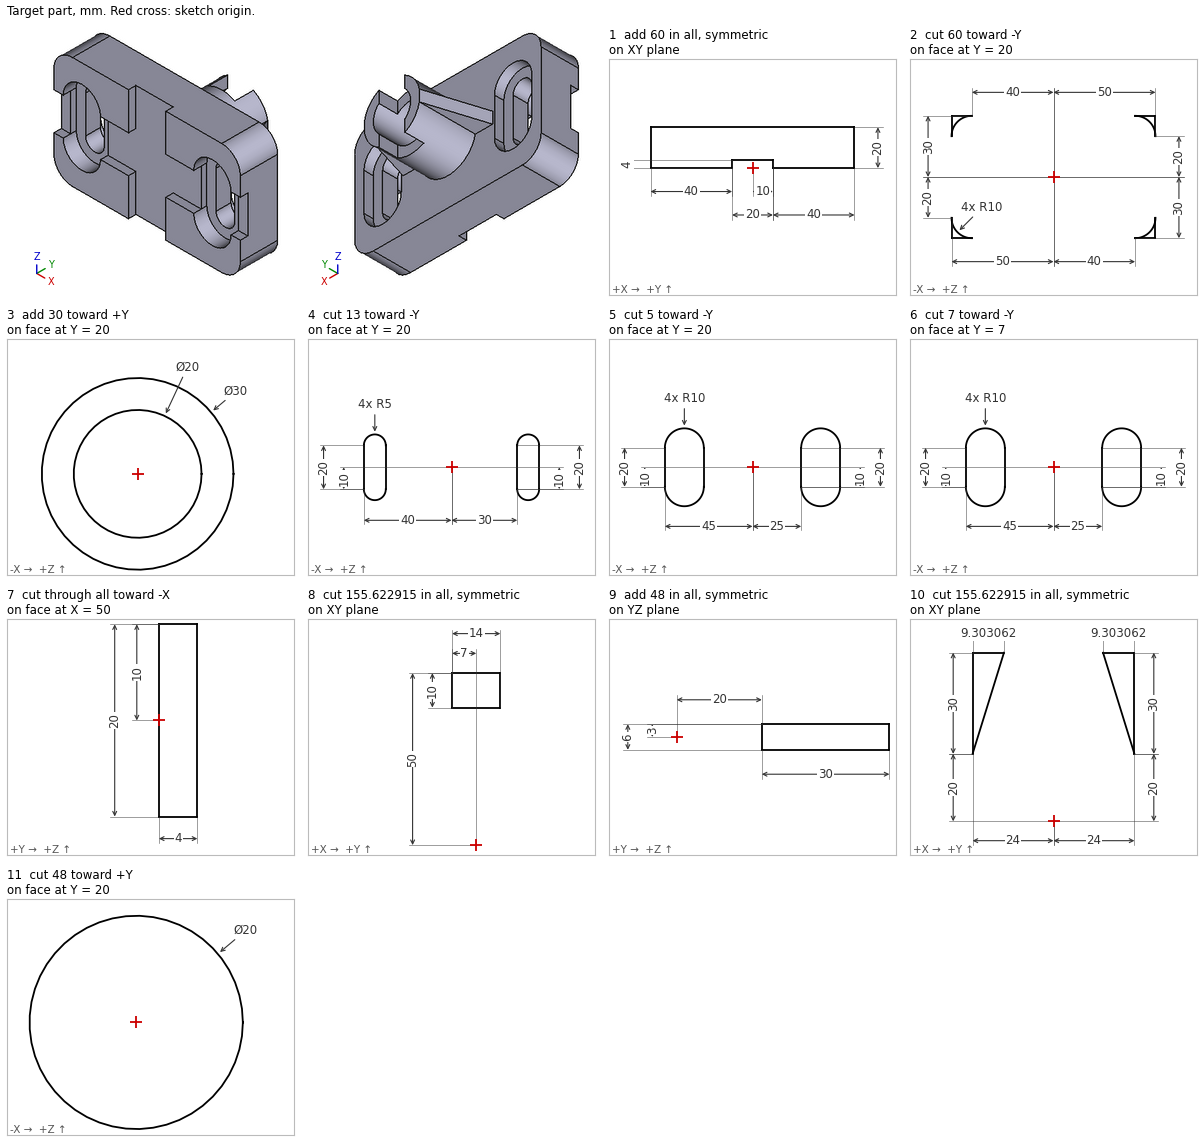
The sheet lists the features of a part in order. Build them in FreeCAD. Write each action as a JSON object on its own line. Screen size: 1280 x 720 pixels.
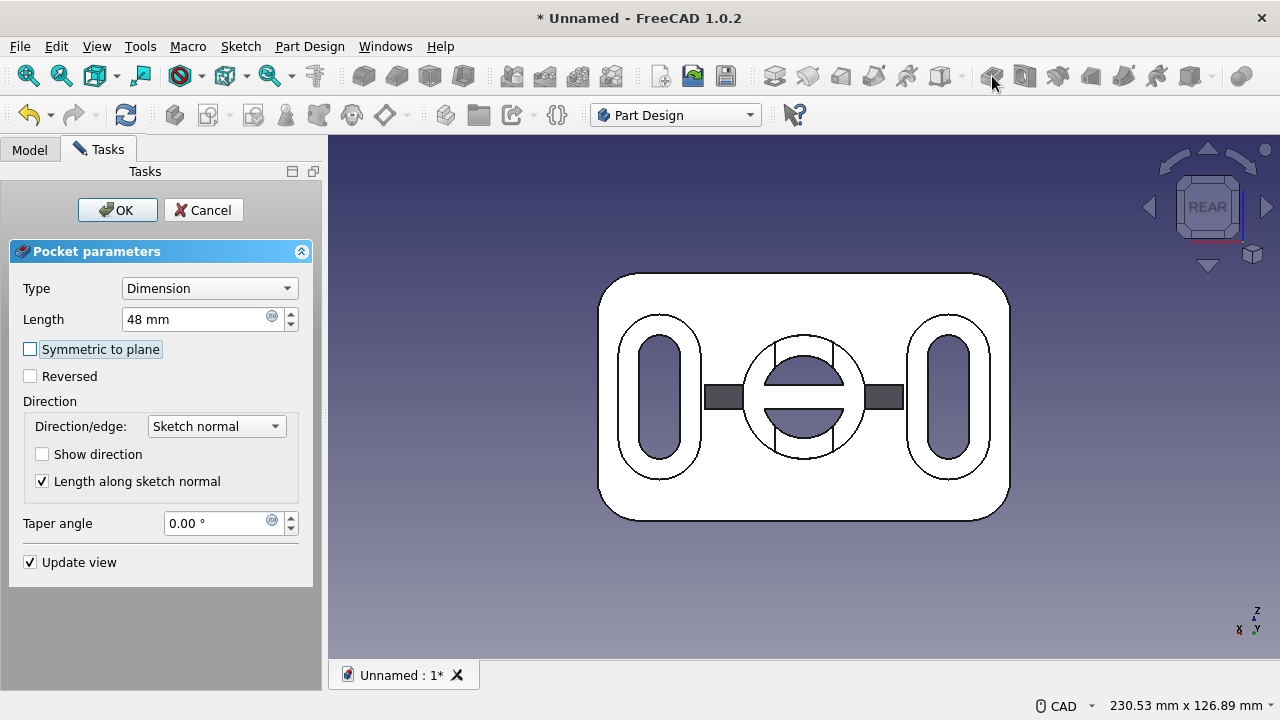
{"action": "left_click", "coordinate": [31, 376]}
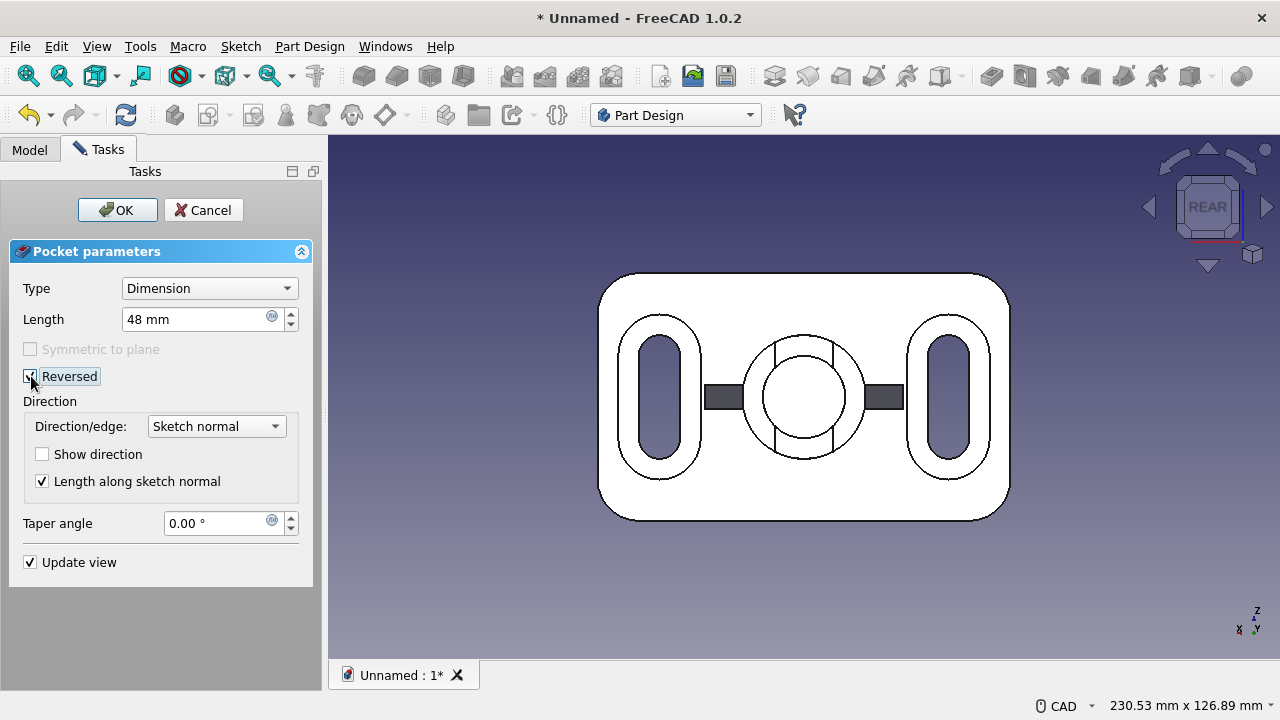
{"action": "left_click", "coordinate": [118, 210]}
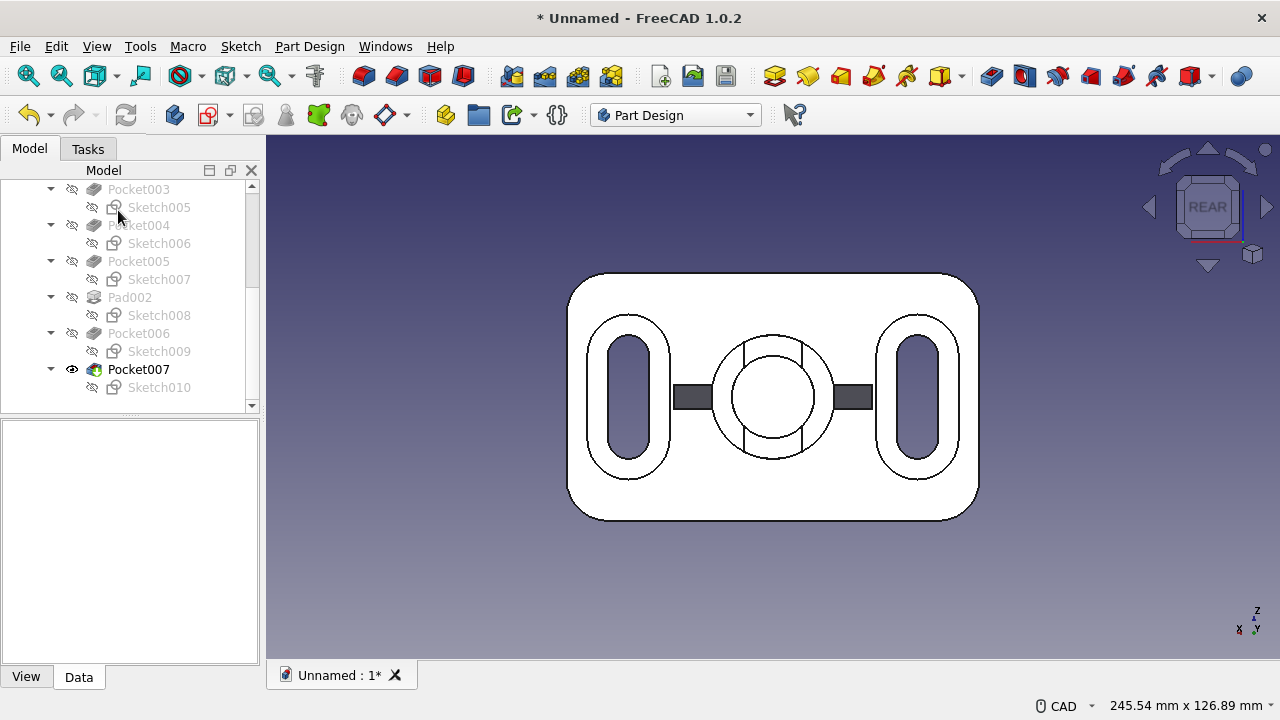
{"action": "key", "text": "0"}